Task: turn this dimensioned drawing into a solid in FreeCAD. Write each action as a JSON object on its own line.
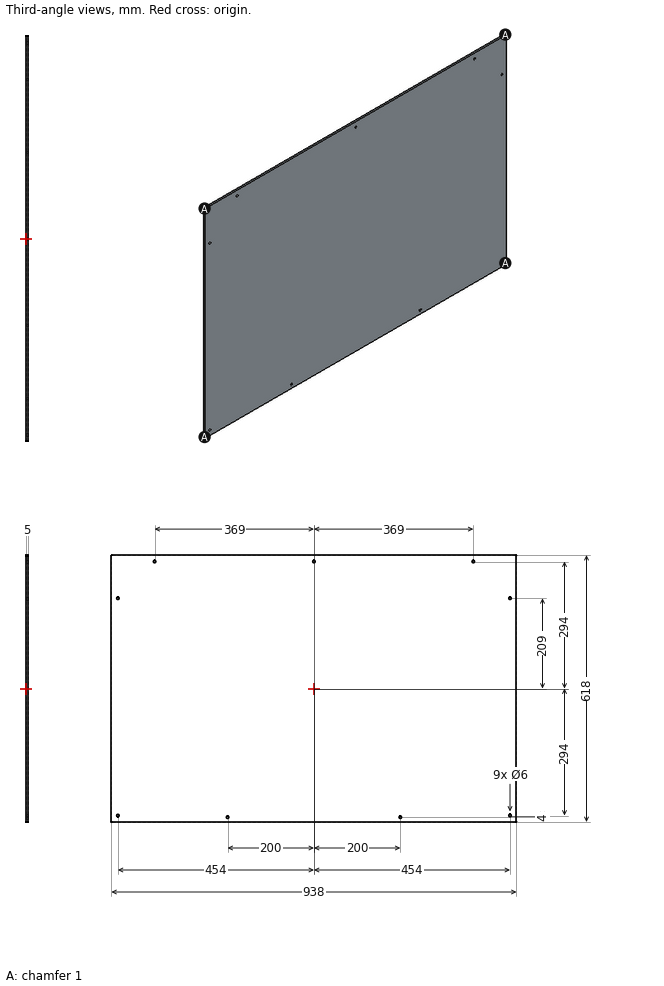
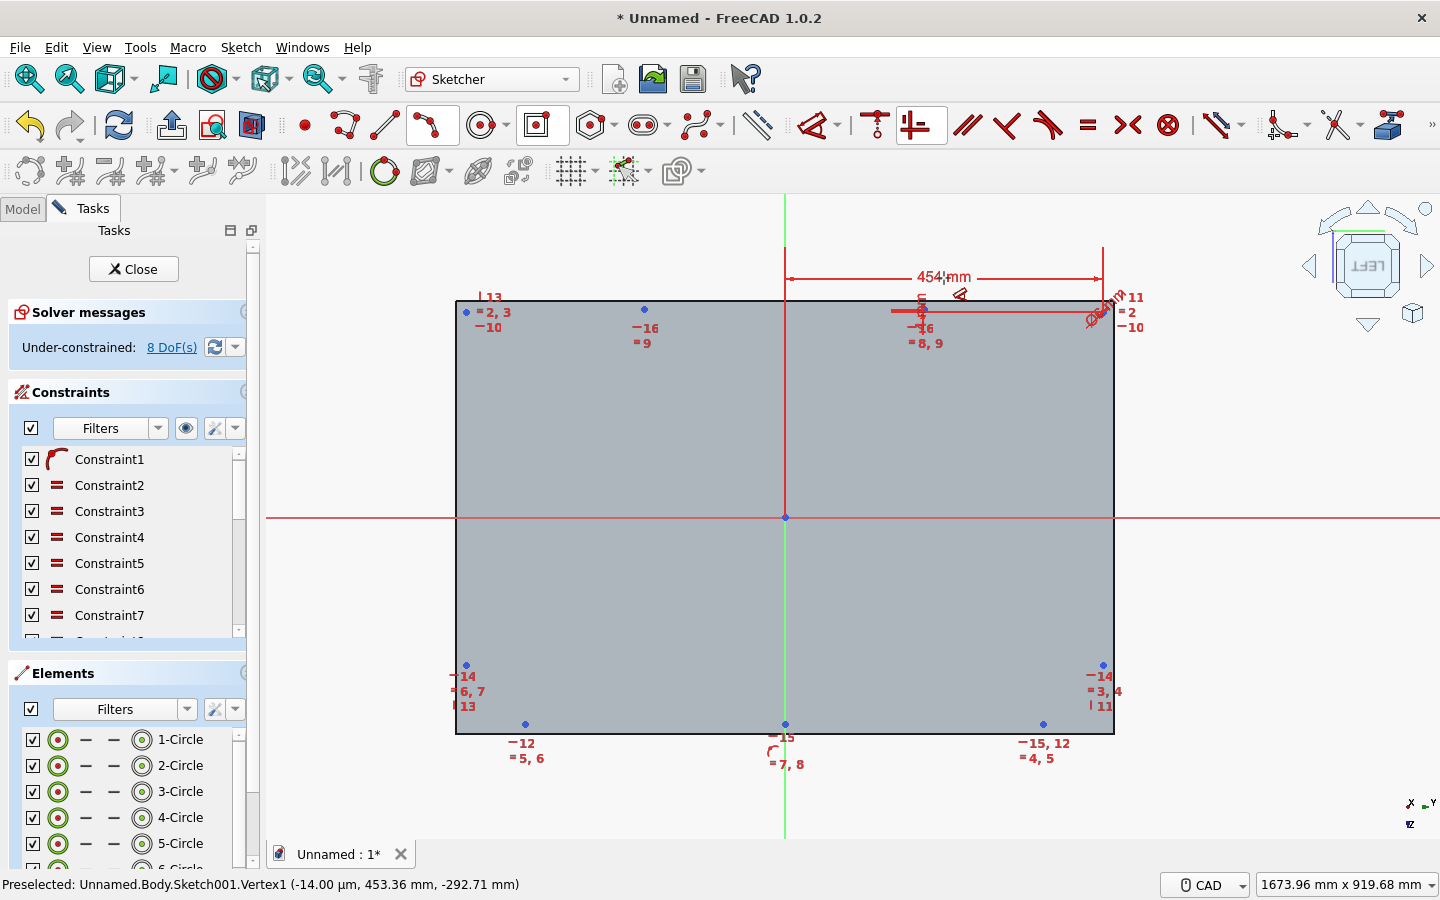
{"action": "left_click", "coordinate": [1103, 312]}
{"action": "left_click", "coordinate": [1137, 415]}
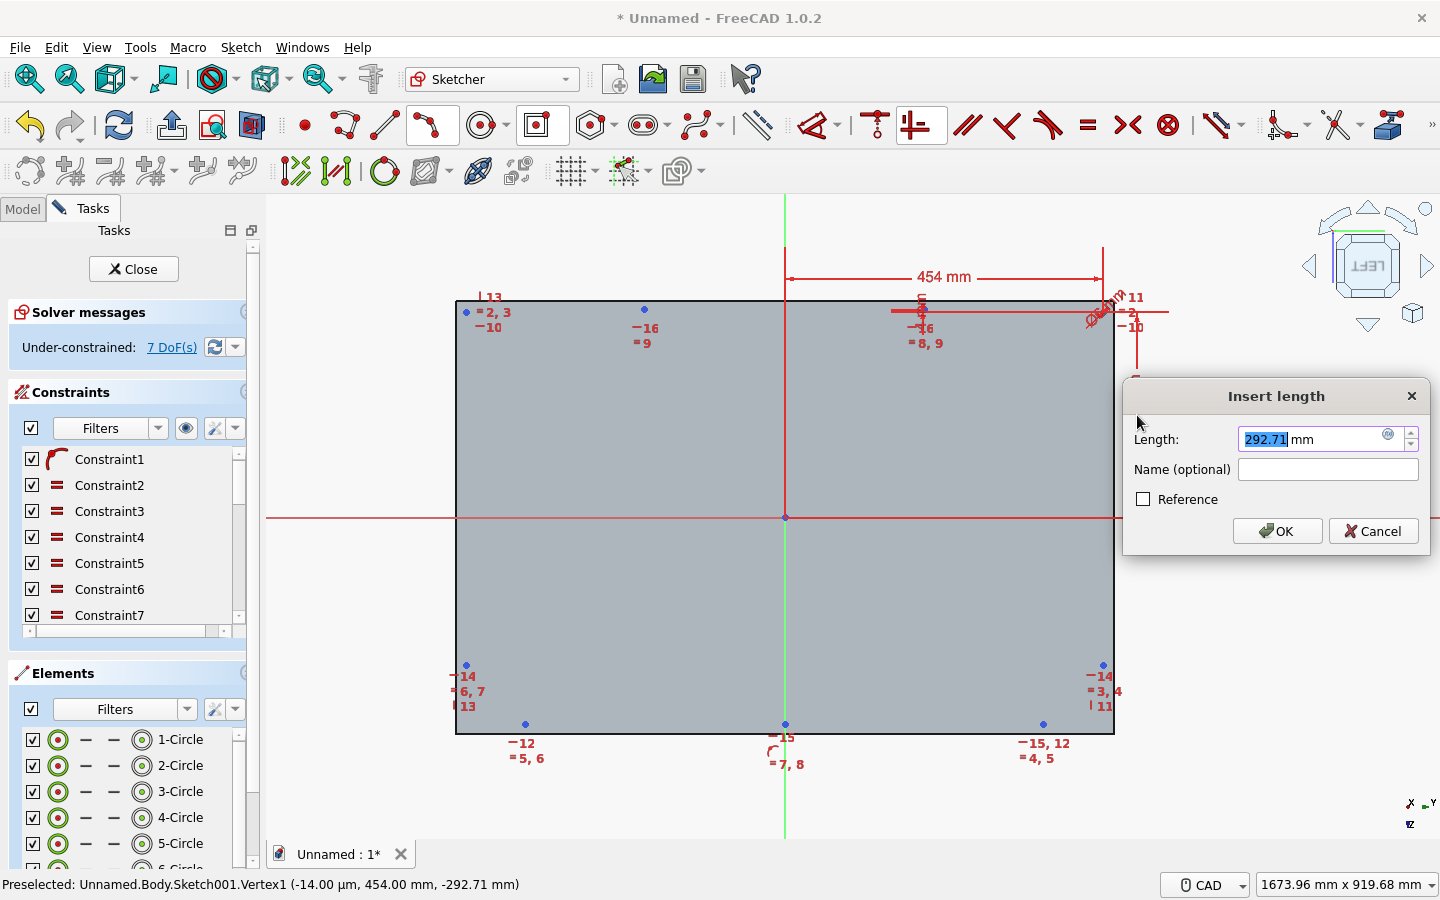
{"action": "type", "text": "294"}
{"action": "key", "text": "Return"}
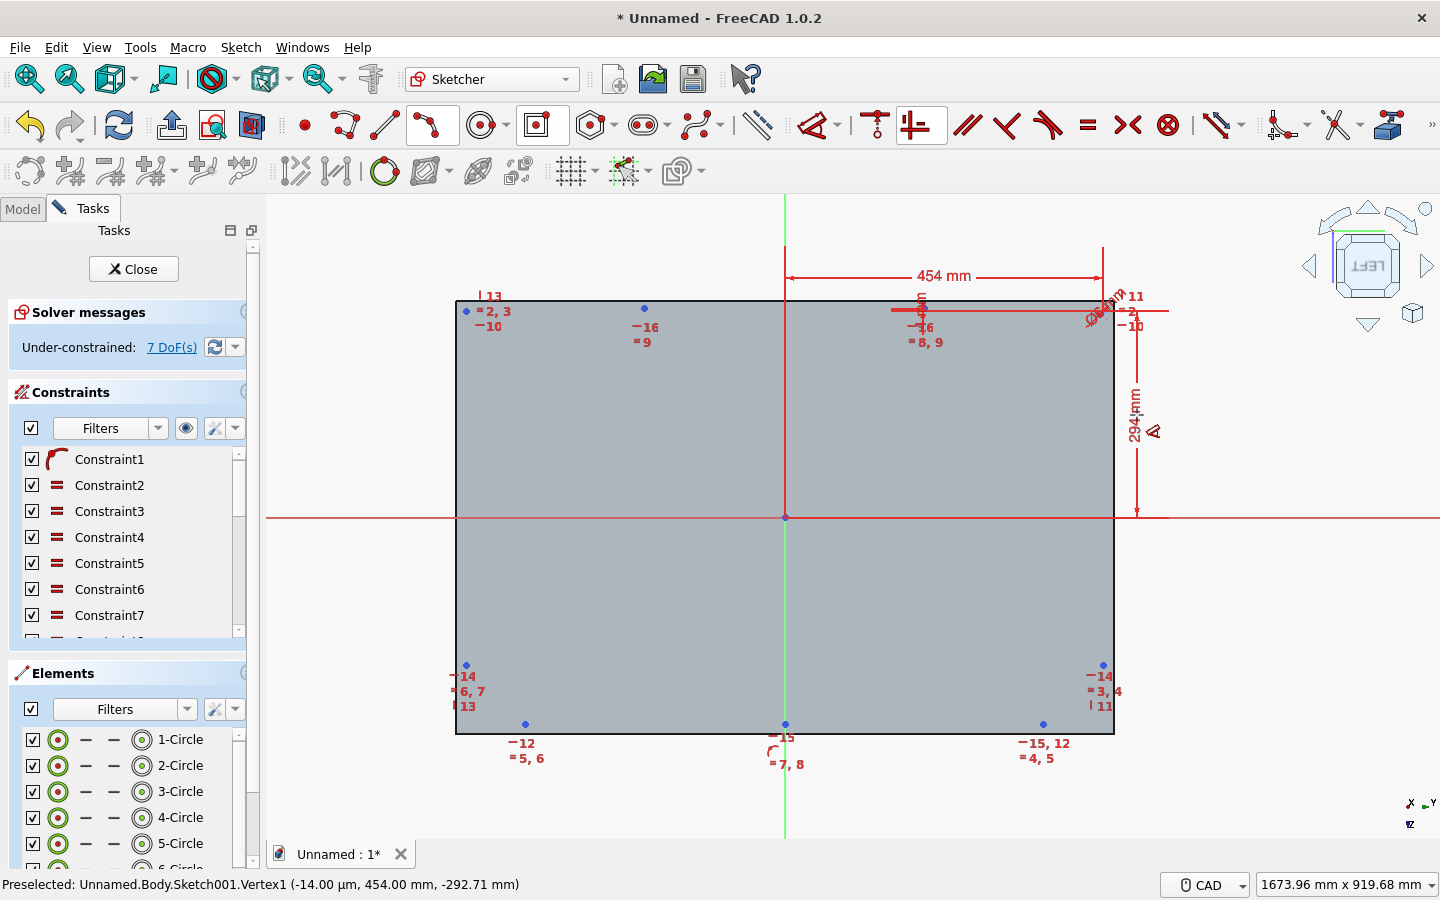
{"action": "left_click", "coordinate": [467, 311]}
{"action": "left_click", "coordinate": [626, 277]}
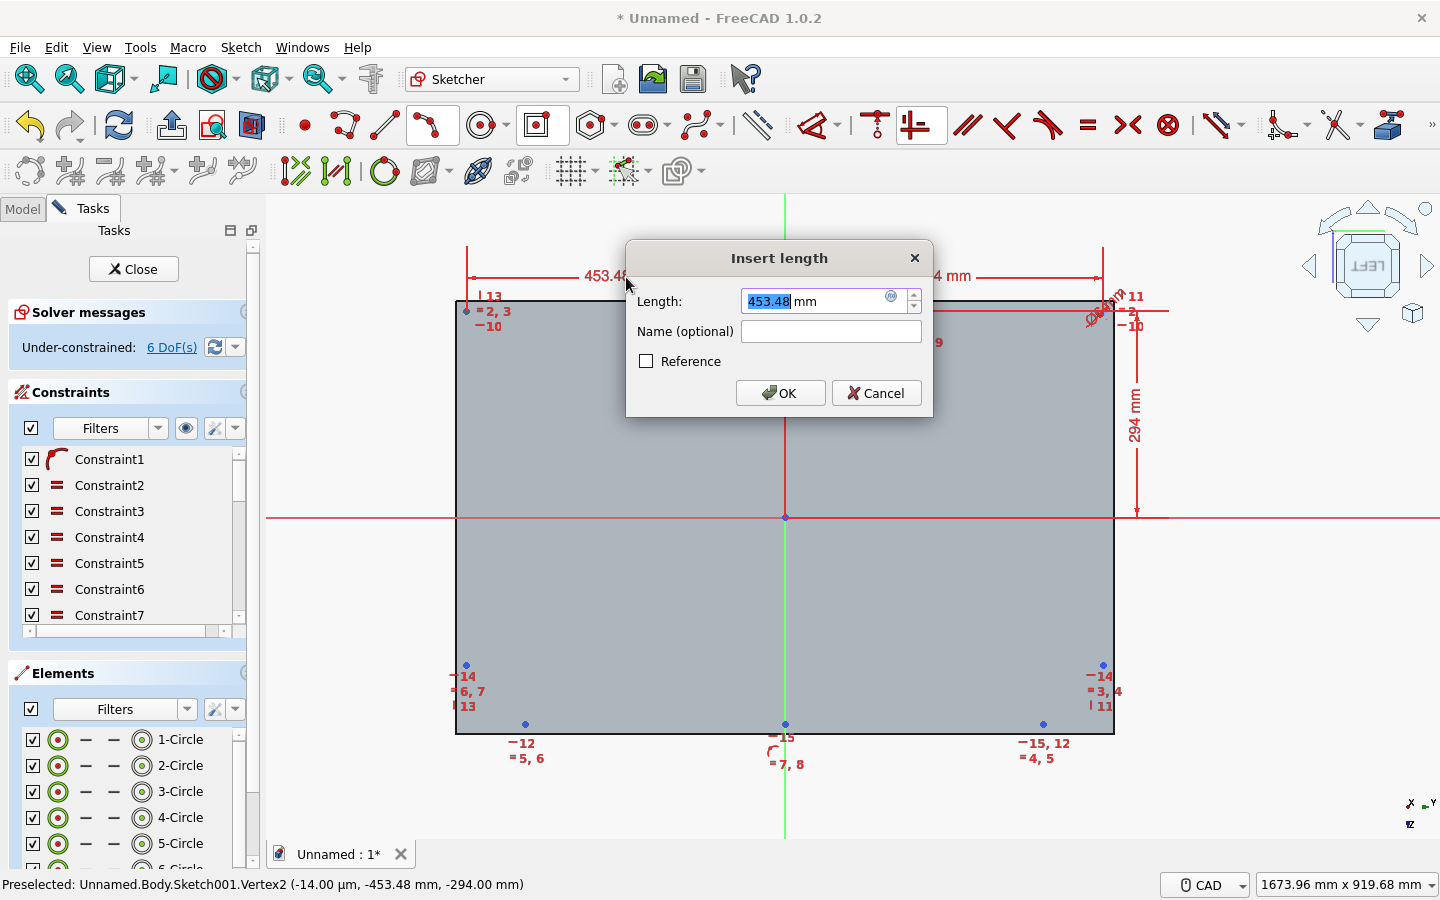
{"action": "type", "text": "454"}
{"action": "key", "text": "Return"}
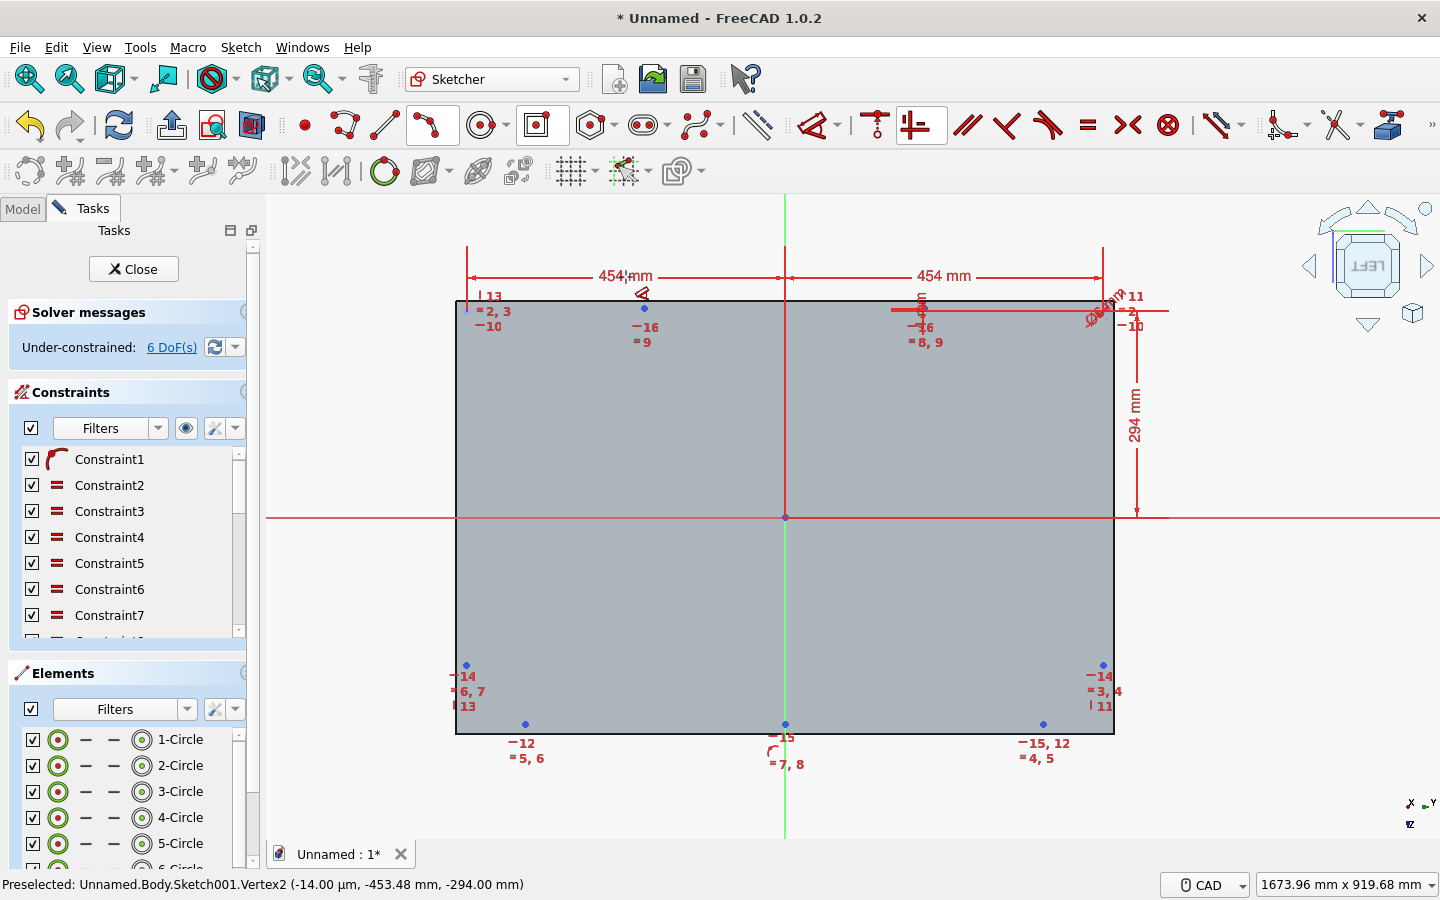
{"action": "left_click", "coordinate": [1103, 665]}
{"action": "left_click", "coordinate": [1137, 592]}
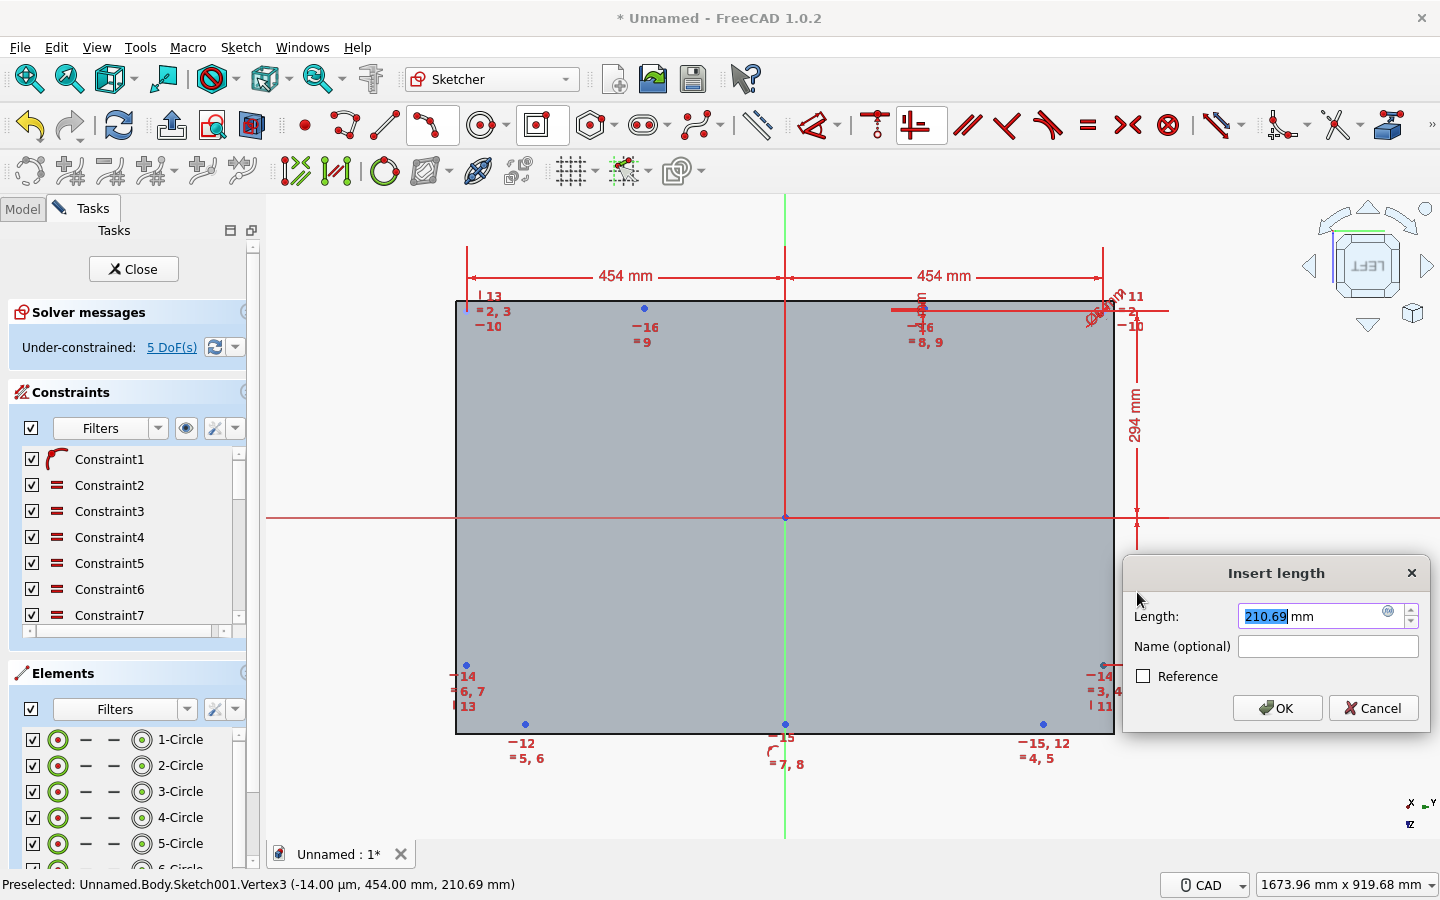
{"action": "type", "text": "209"}
{"action": "key", "text": "Return"}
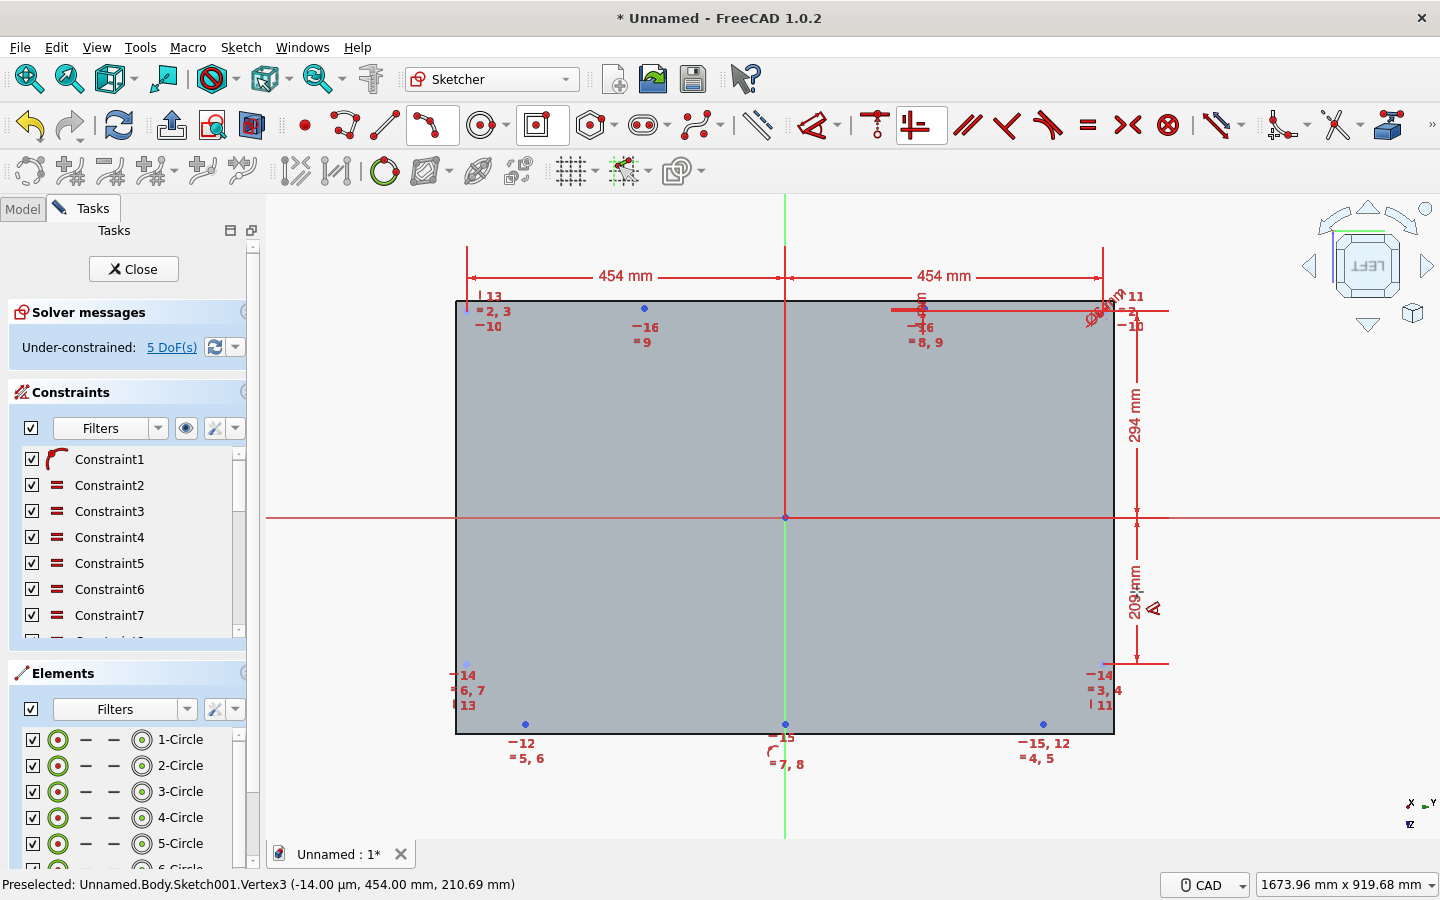
{"action": "left_click", "coordinate": [1044, 724]}
{"action": "left_click", "coordinate": [914, 758]}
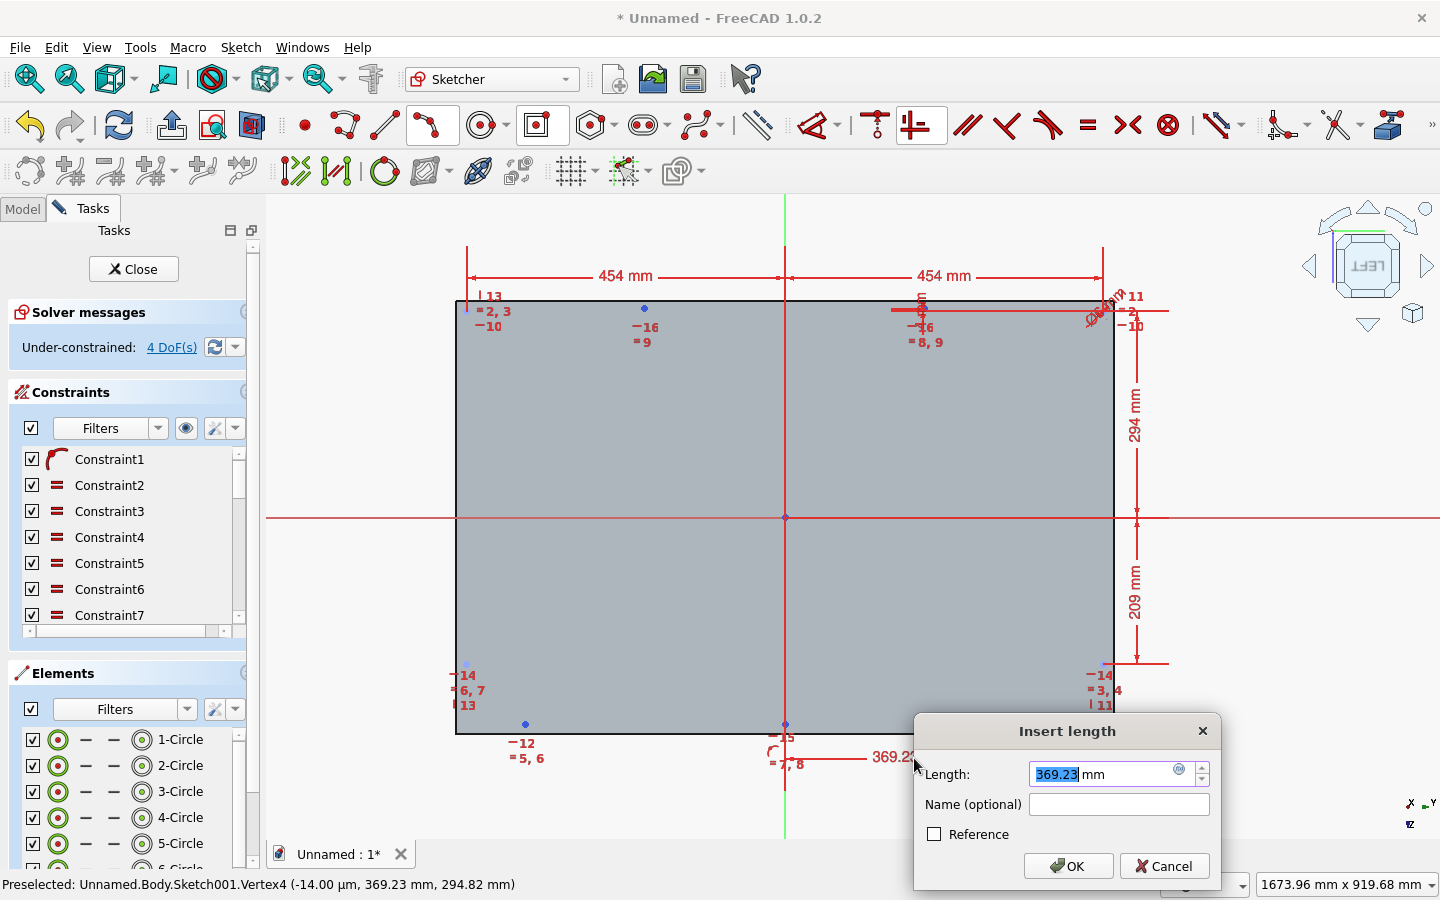
{"action": "type", "text": "369"}
{"action": "key", "text": "Return"}